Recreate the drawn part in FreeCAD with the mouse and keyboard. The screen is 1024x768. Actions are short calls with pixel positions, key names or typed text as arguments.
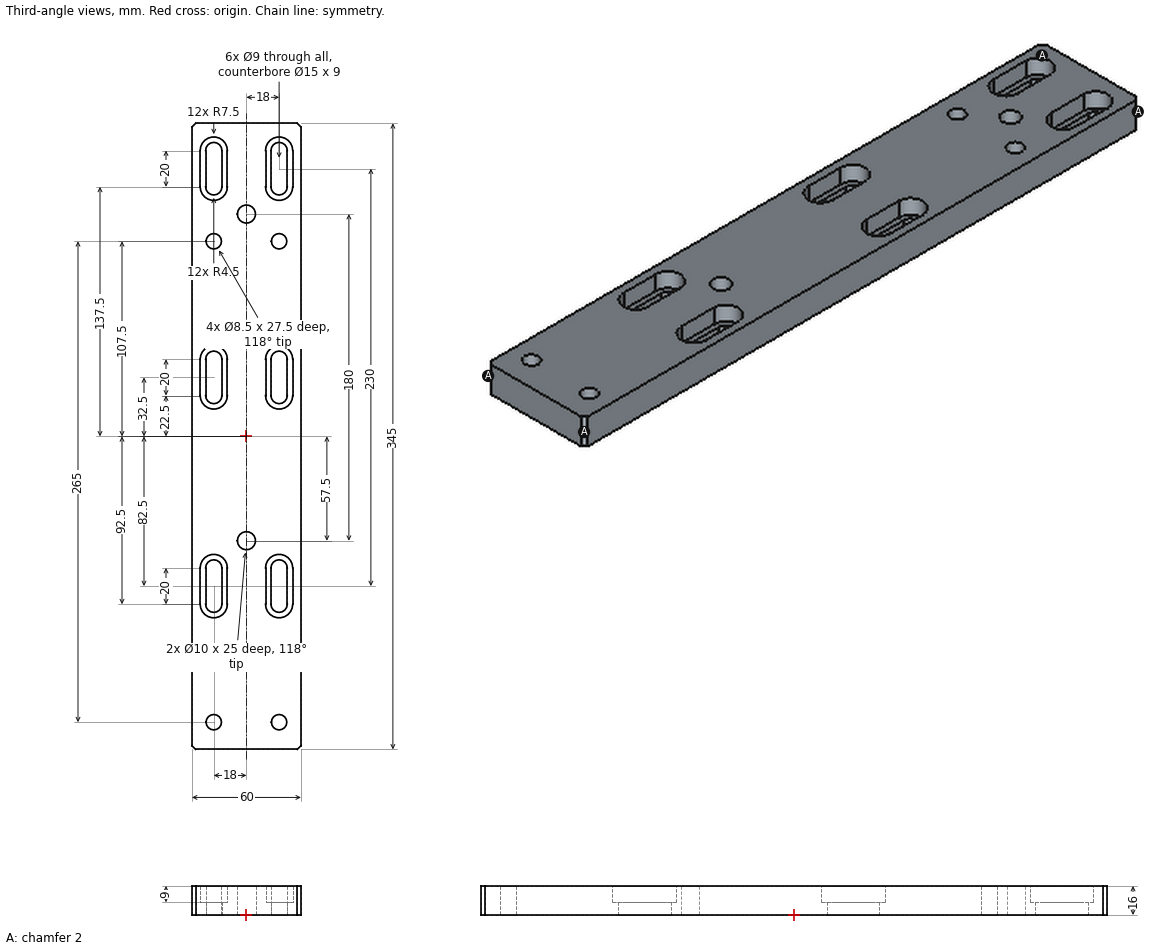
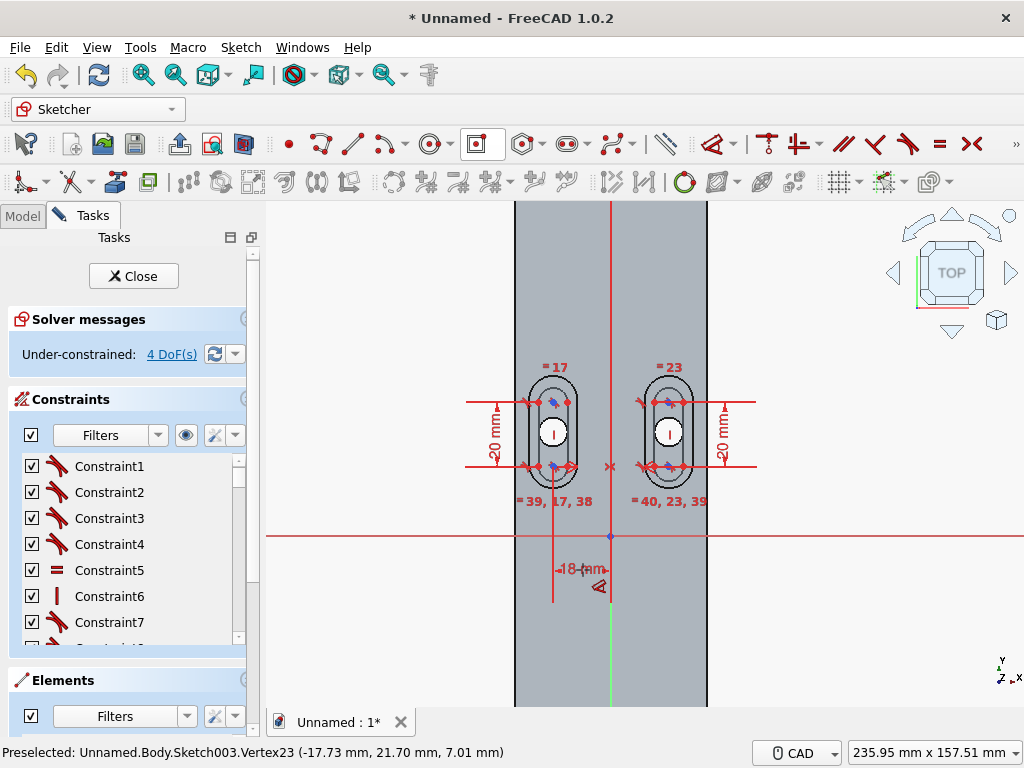
scroll(556, 467, down, 5)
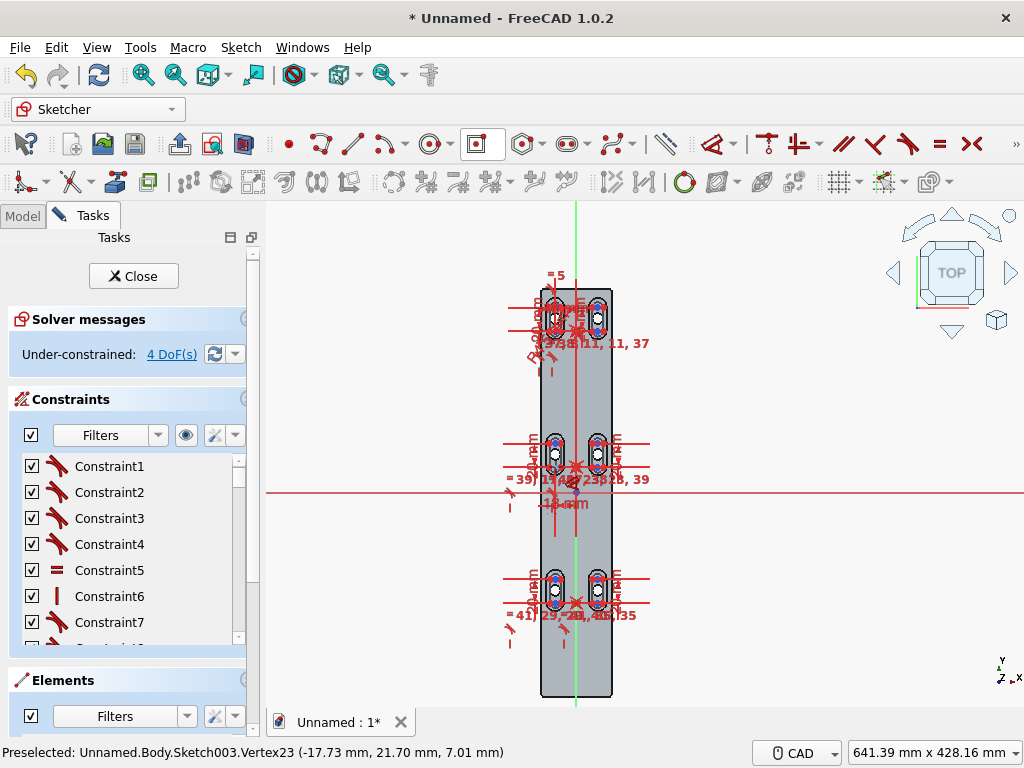
scroll(555, 603, up, 5)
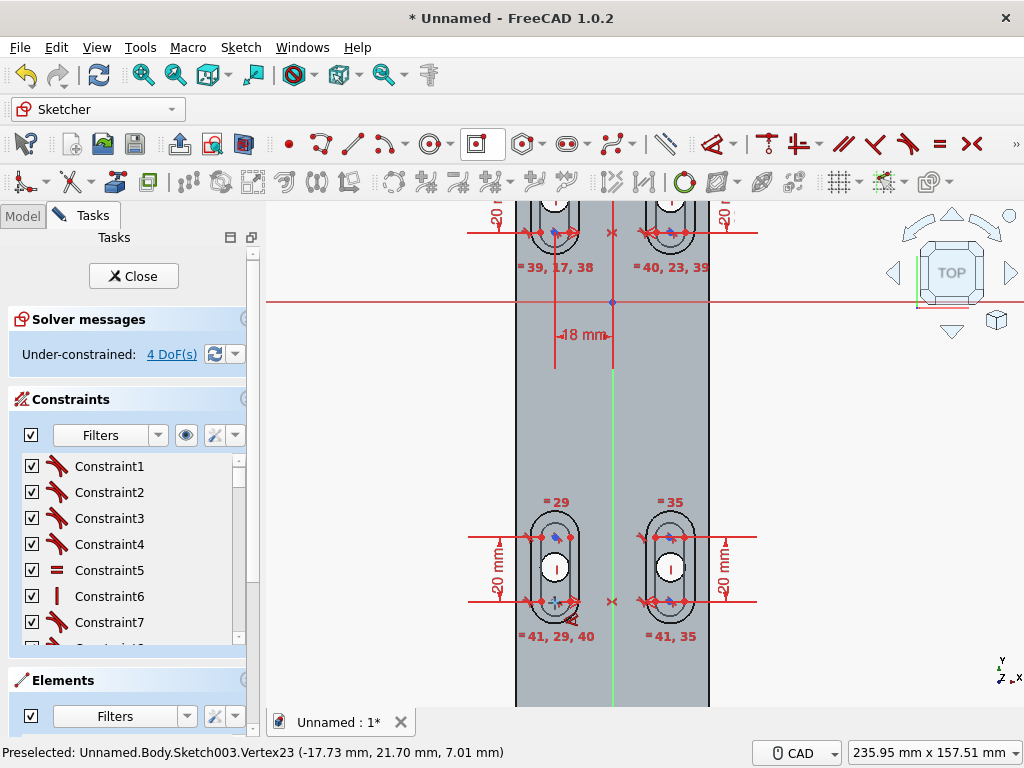
click(556, 602)
click(584, 636)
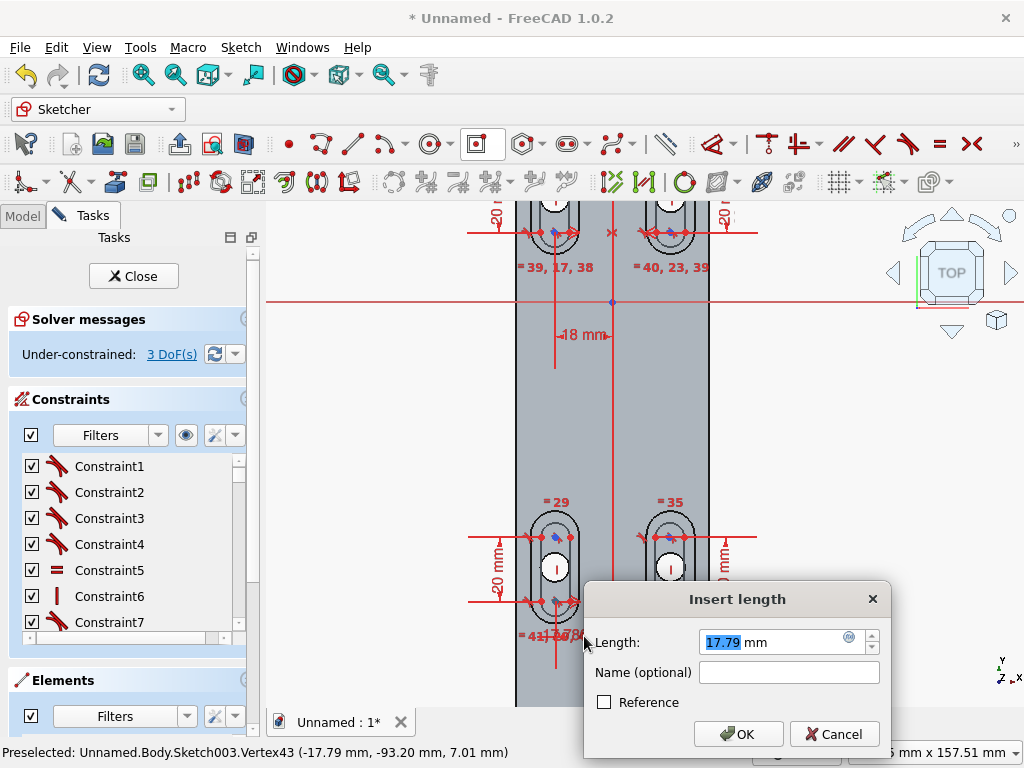
text(18)
key(Return)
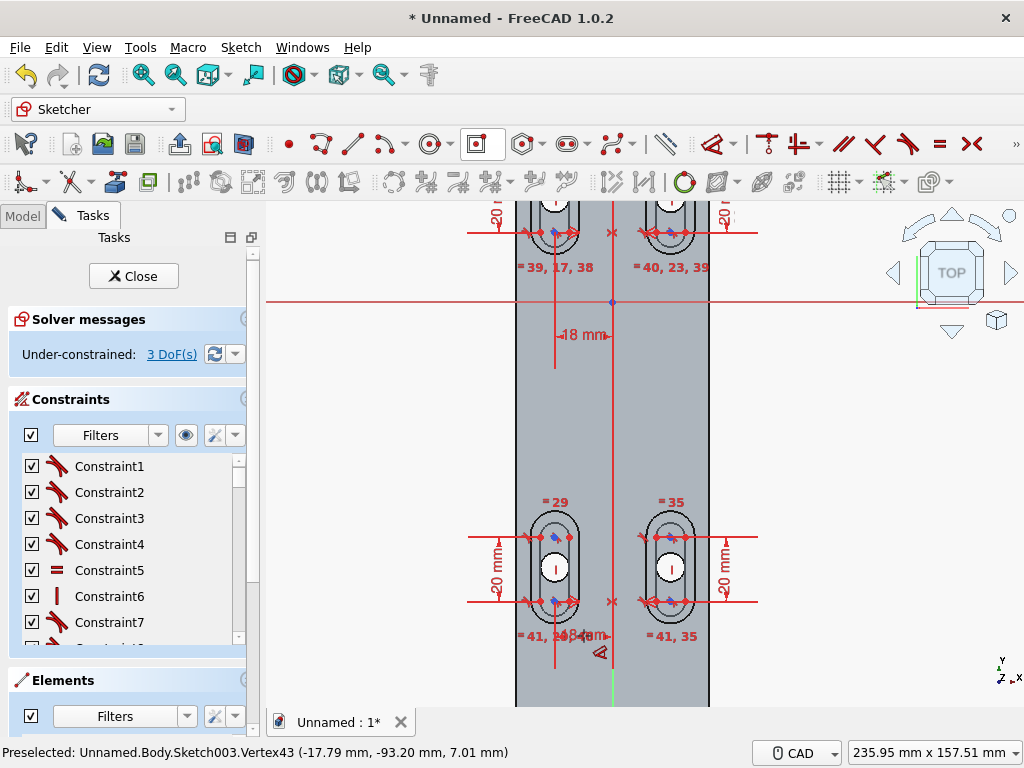
click(540, 233)
click(506, 267)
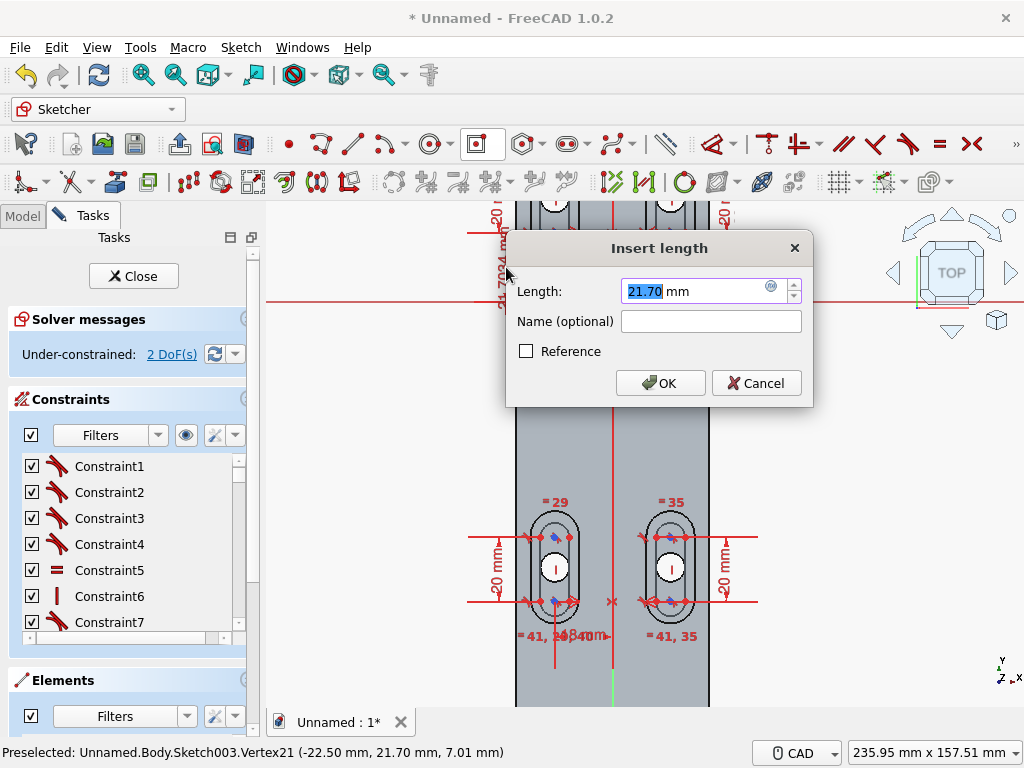
text(22.5)
key(Return)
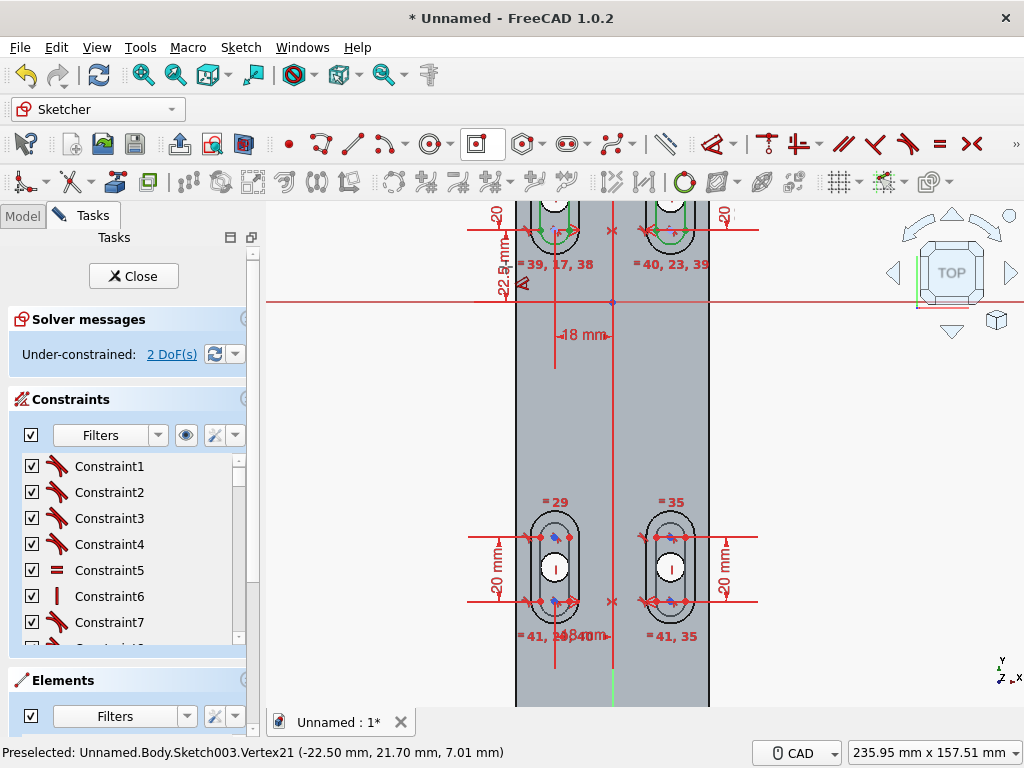
click(540, 602)
click(506, 452)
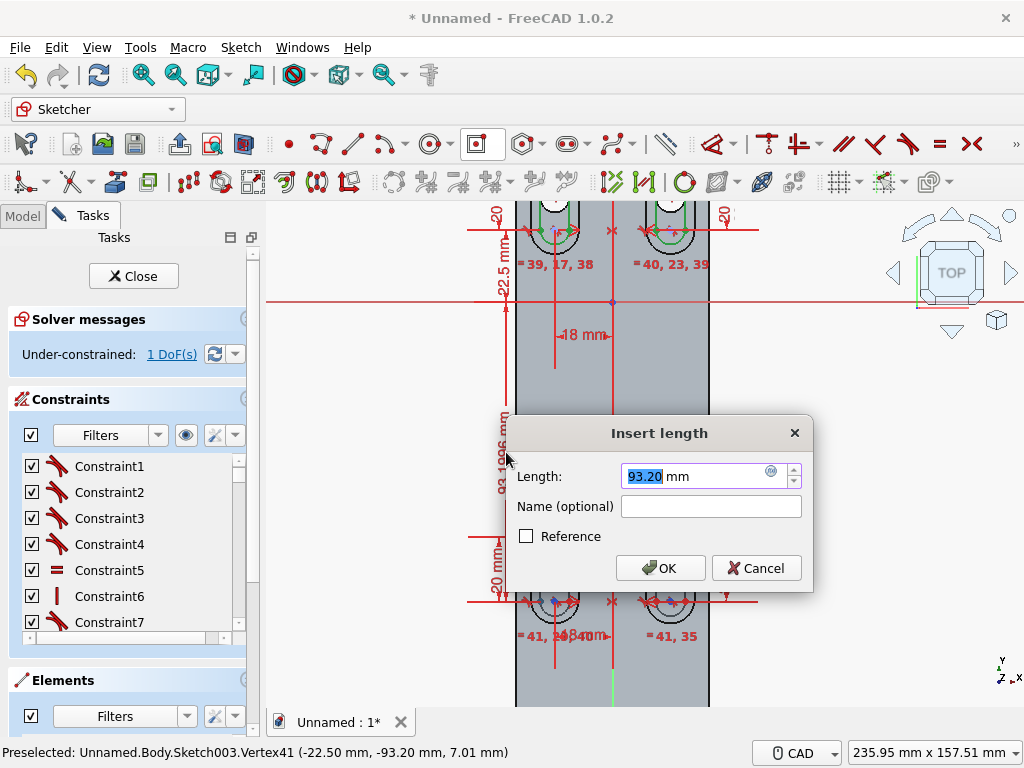
text(92.5)
key(Return)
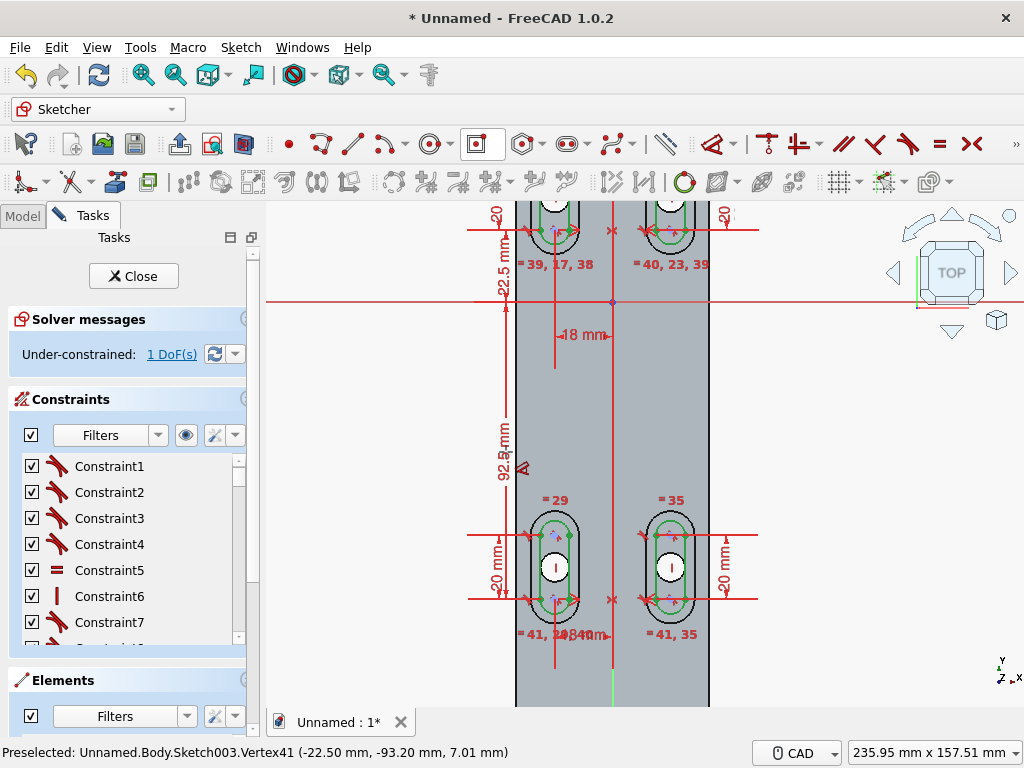
scroll(555, 603, down, 5)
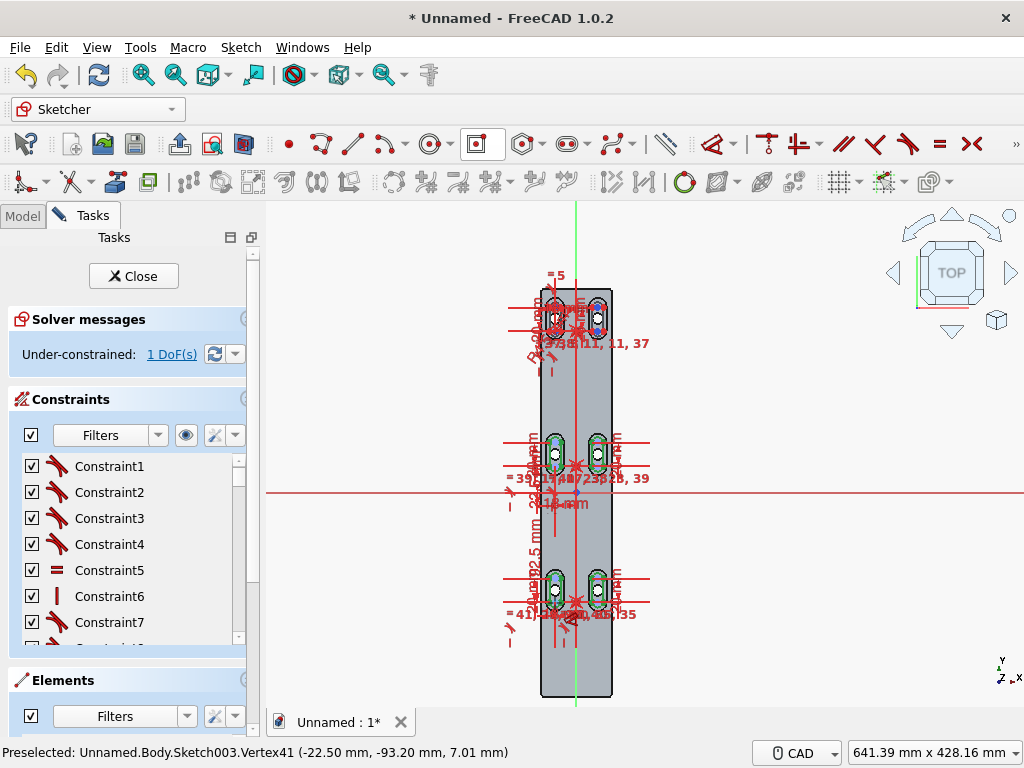
scroll(550, 331, up, 5)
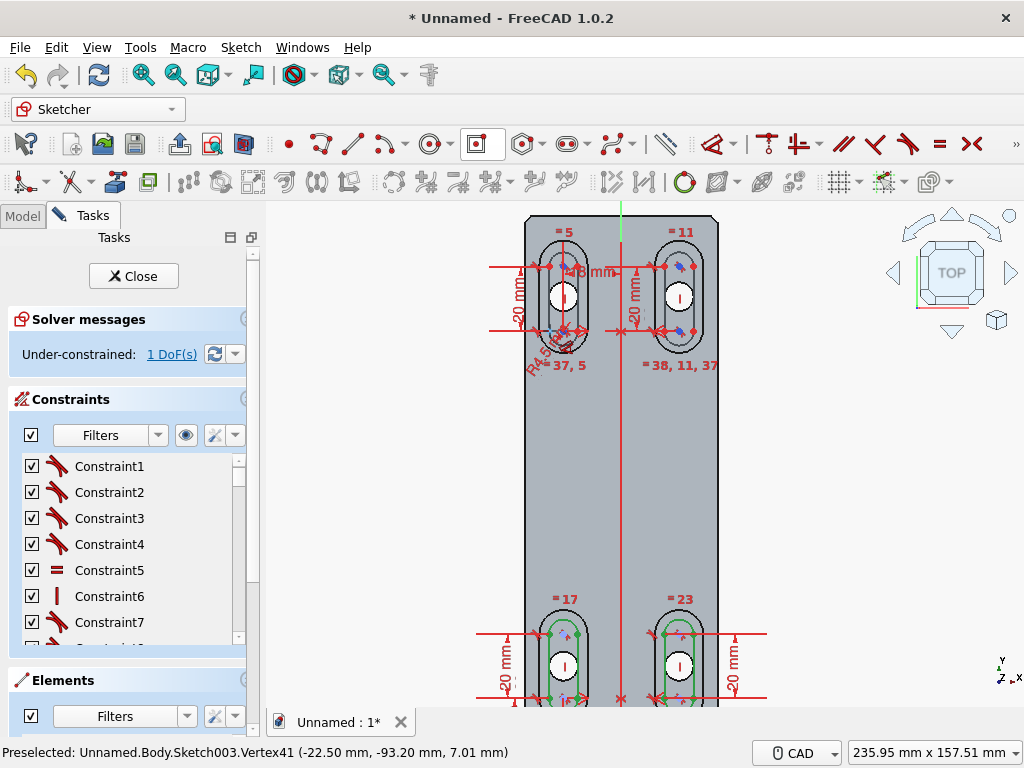
click(549, 331)
click(515, 505)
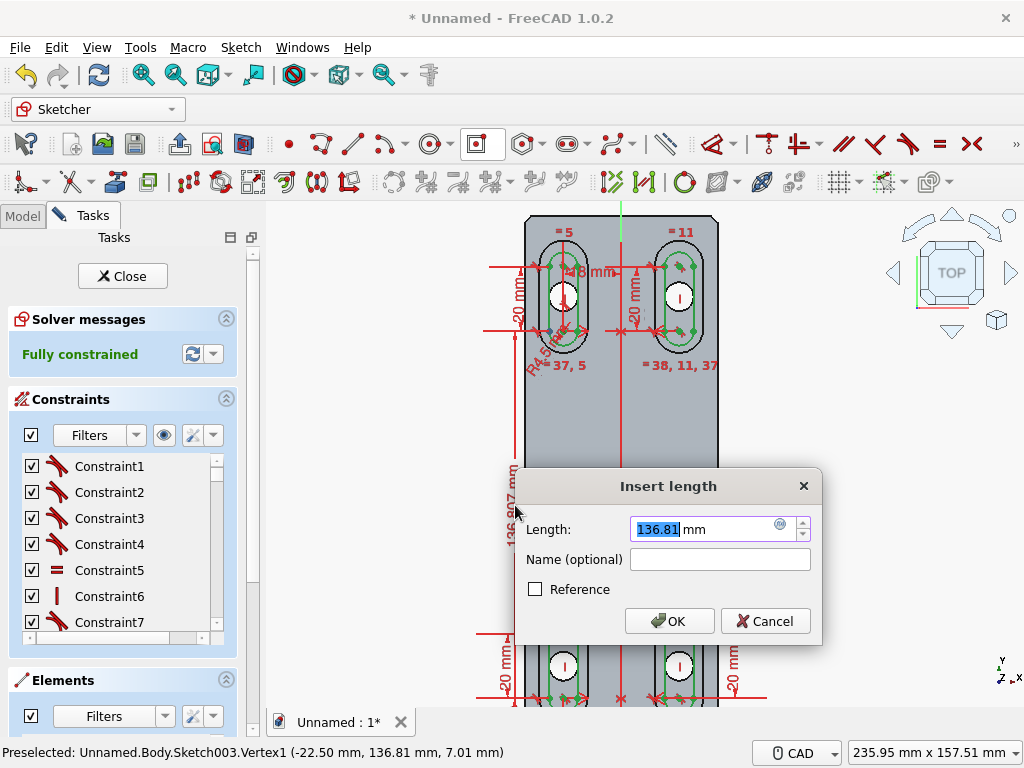
text(137.5)
key(Return)
key(Escape)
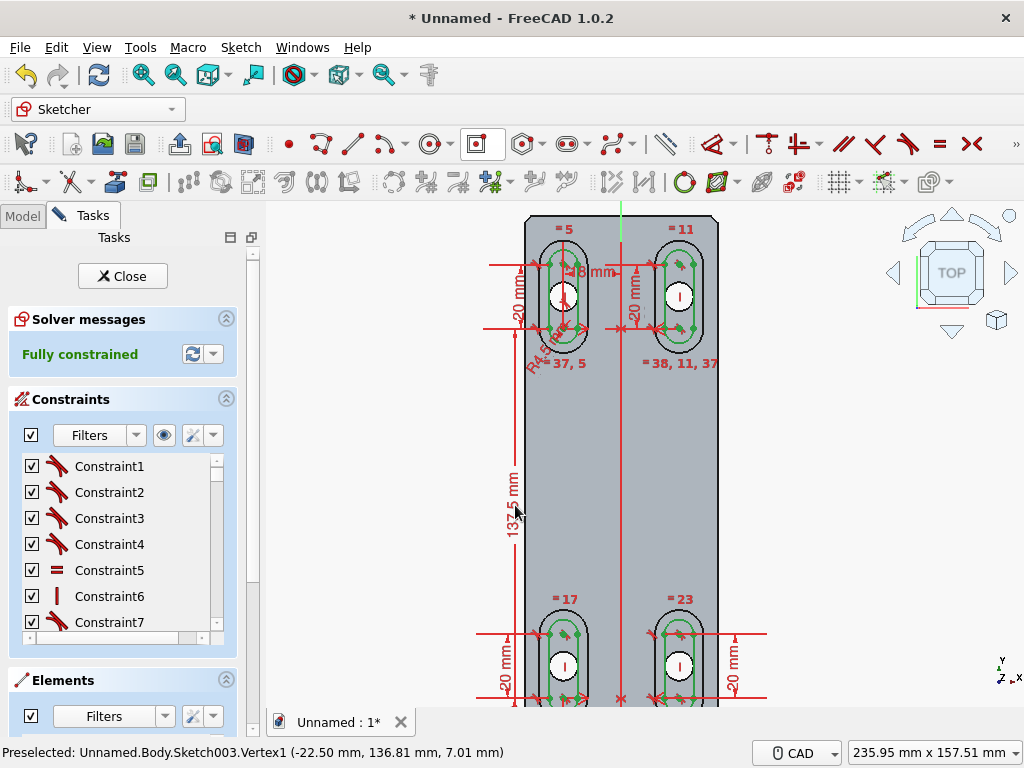
click(123, 276)